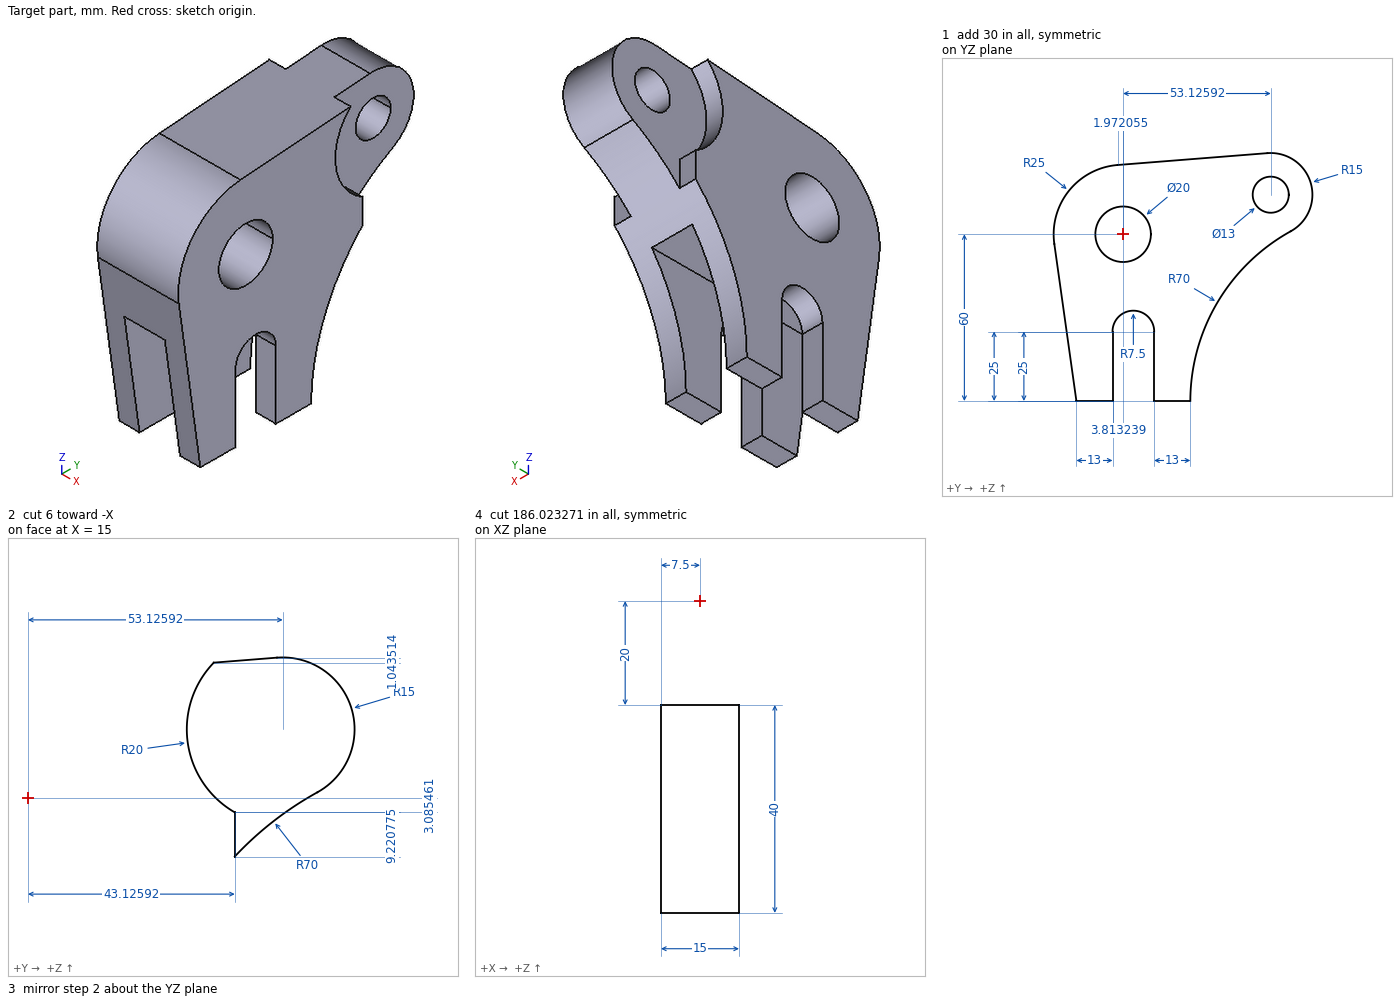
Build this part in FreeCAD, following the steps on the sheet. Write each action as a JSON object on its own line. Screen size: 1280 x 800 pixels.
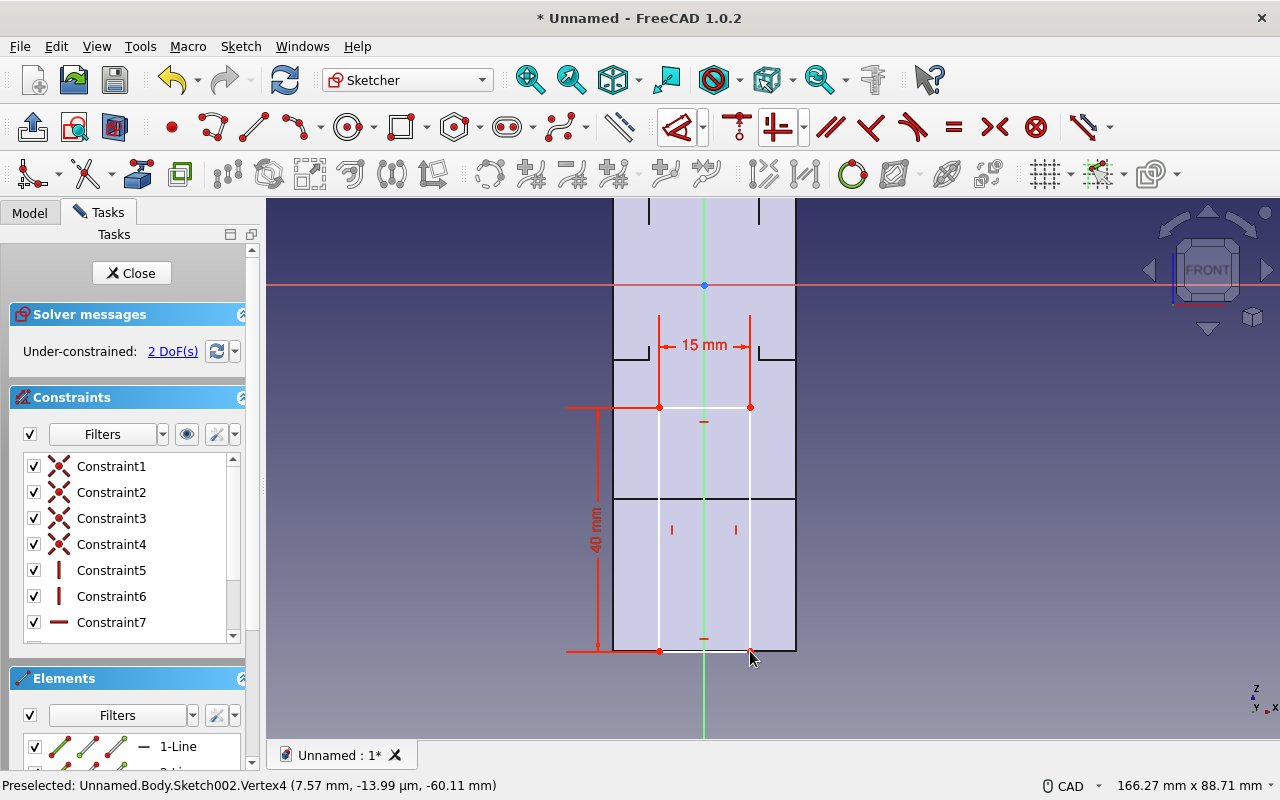
{"action": "left_click", "coordinate": [659, 408]}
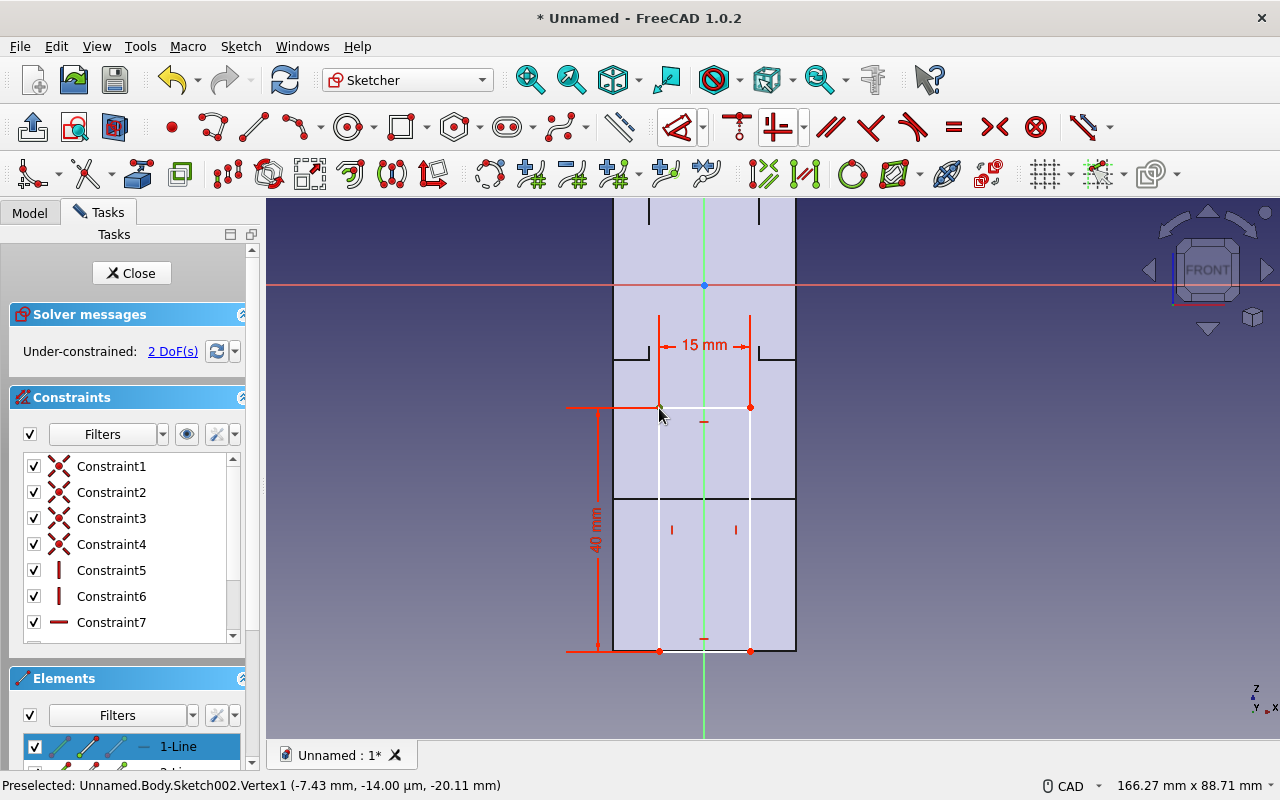
{"action": "left_click", "coordinate": [702, 128]}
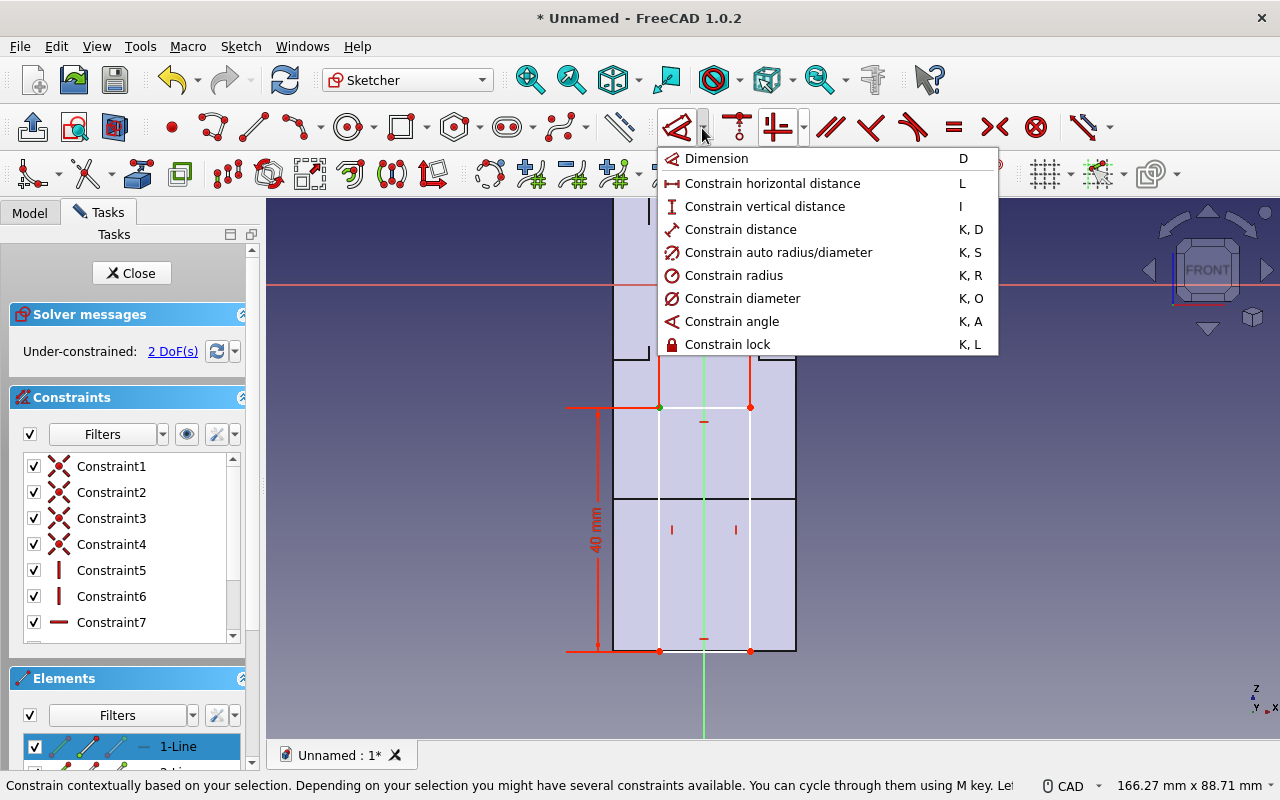
{"action": "left_click", "coordinate": [828, 206]}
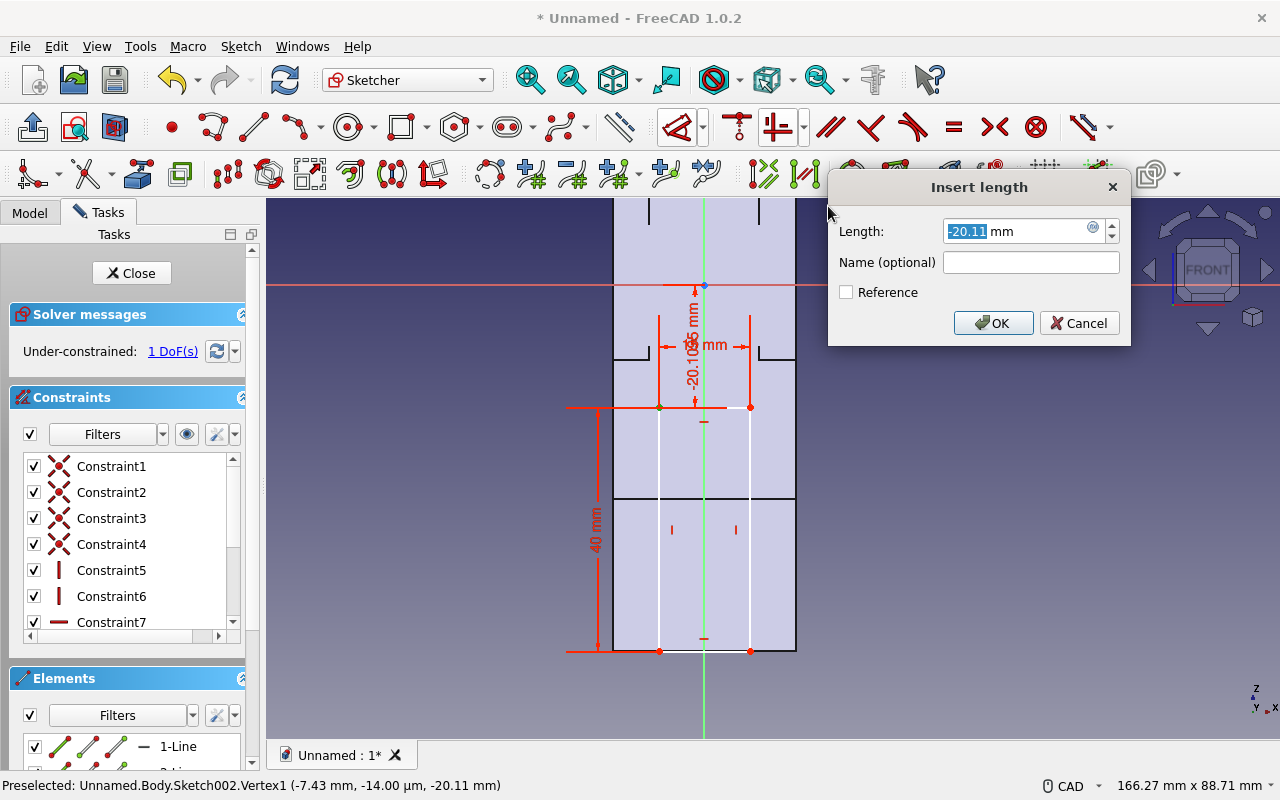
{"action": "type", "text": "-20"}
{"action": "key", "text": "Return"}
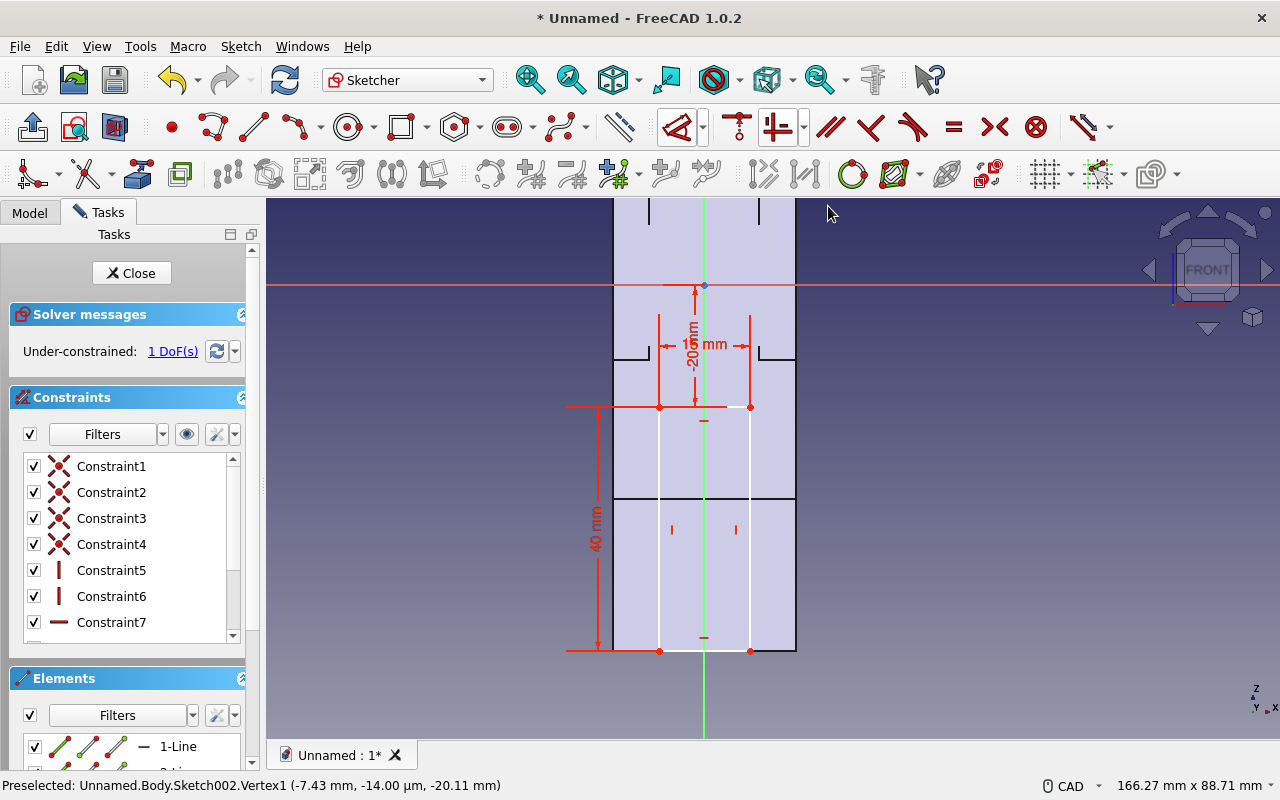
{"action": "left_click", "coordinate": [659, 407]}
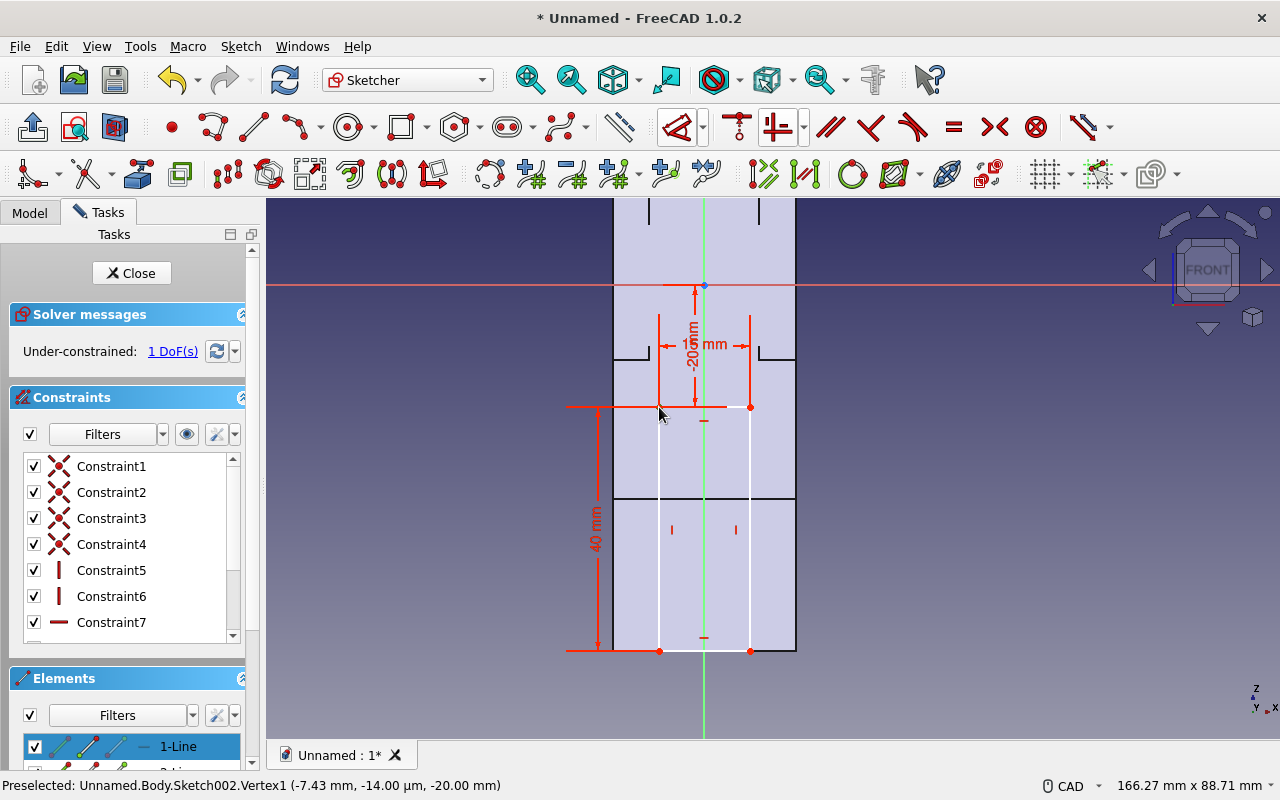
{"action": "key", "text": "l"}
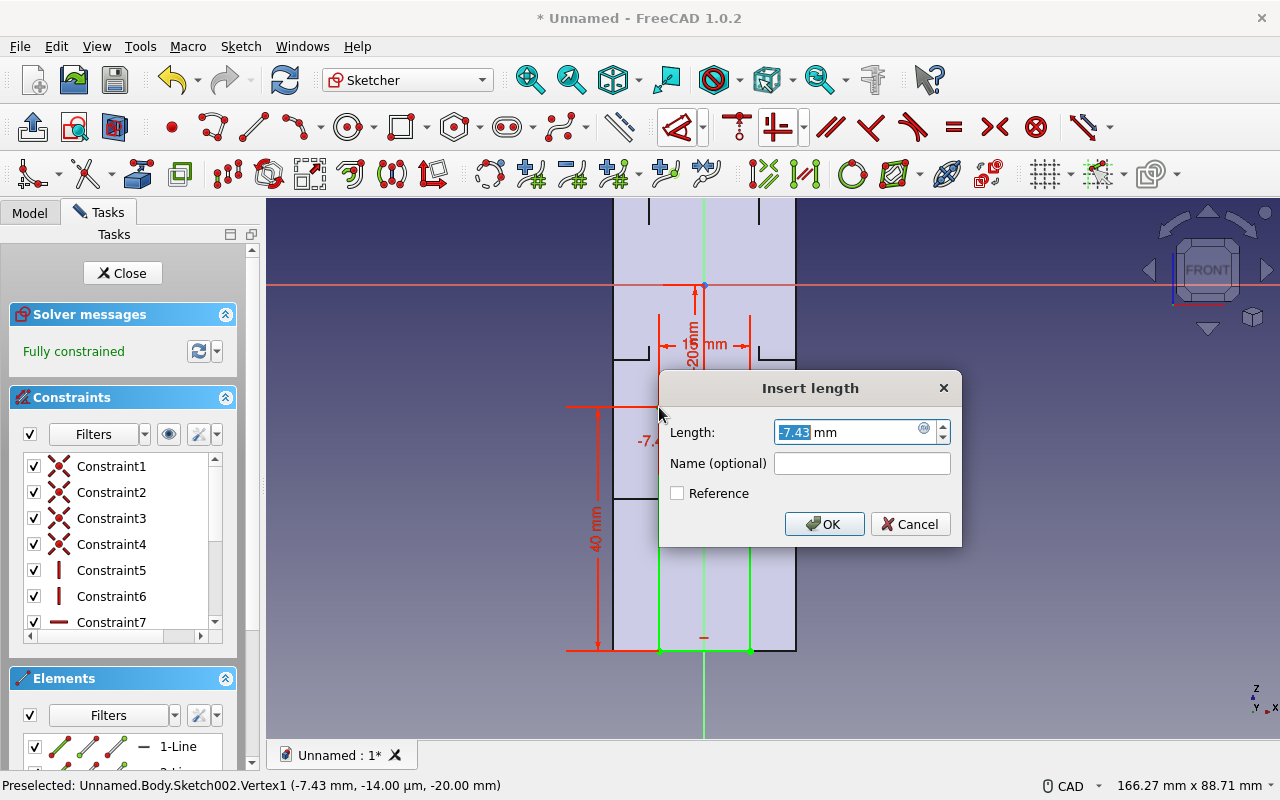
{"action": "type", "text": "-7.5"}
{"action": "key", "text": "Return"}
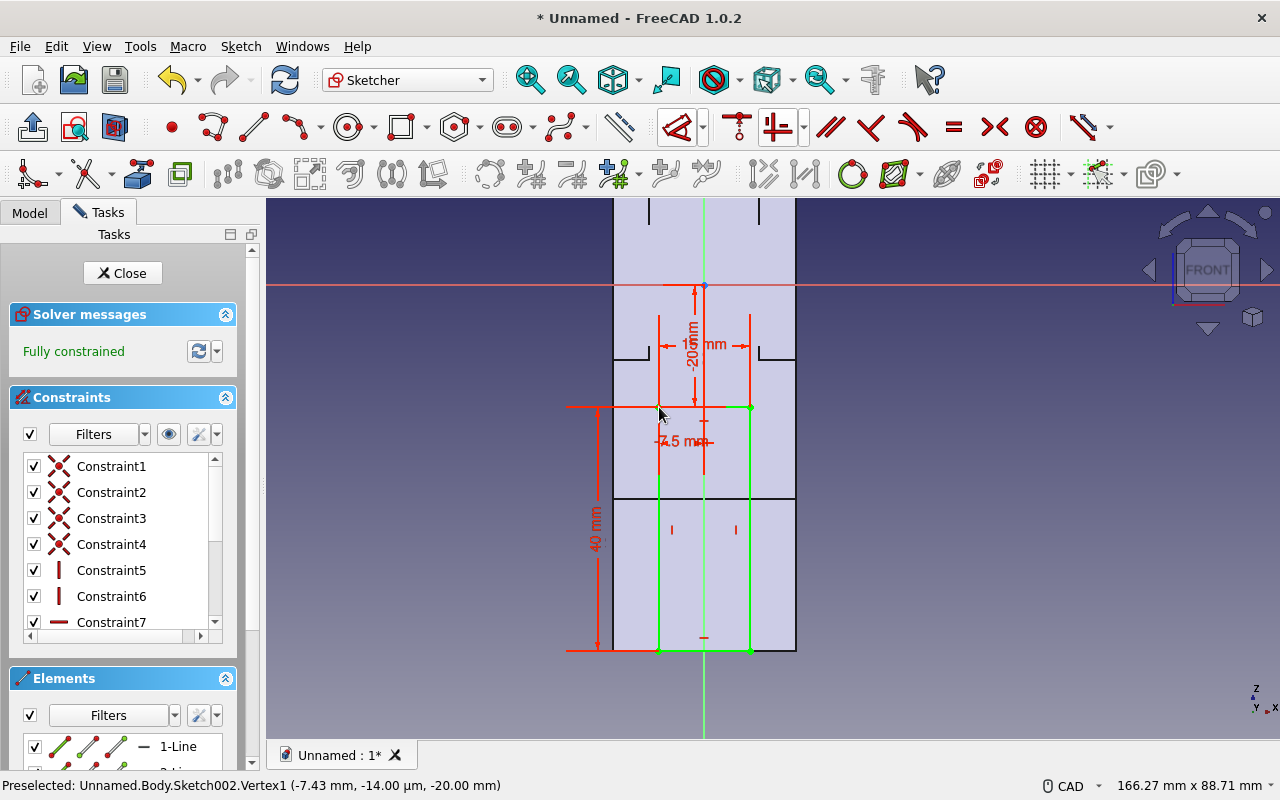
{"action": "left_click", "coordinate": [123, 273]}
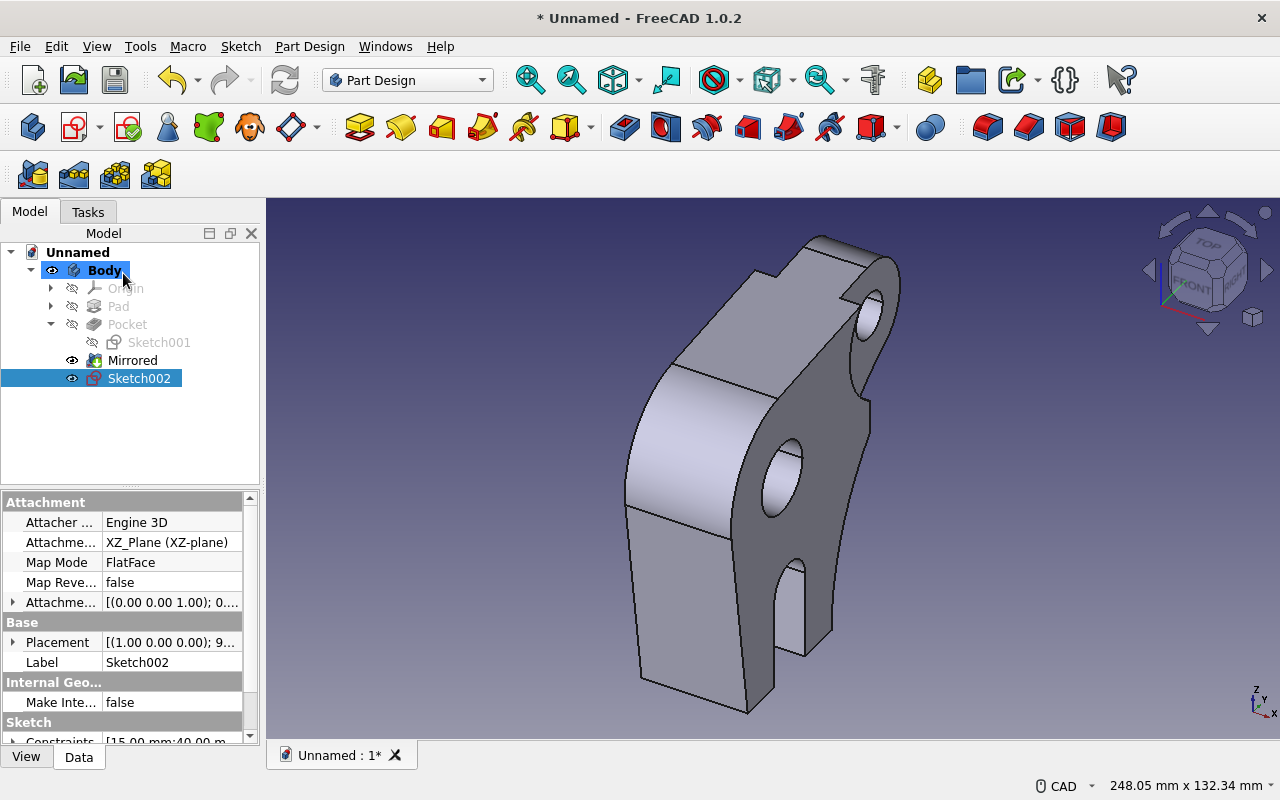
{"action": "left_click", "coordinate": [625, 128]}